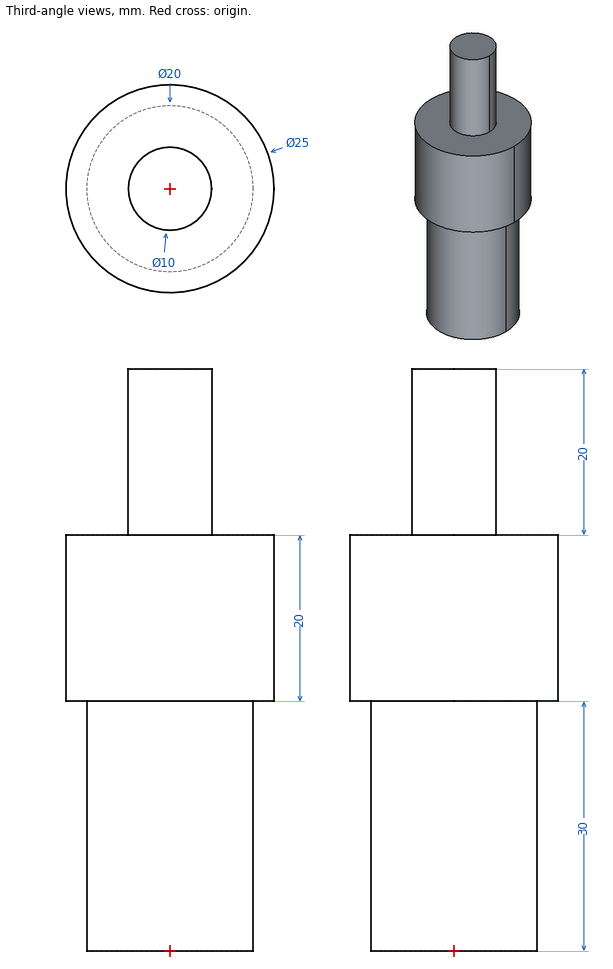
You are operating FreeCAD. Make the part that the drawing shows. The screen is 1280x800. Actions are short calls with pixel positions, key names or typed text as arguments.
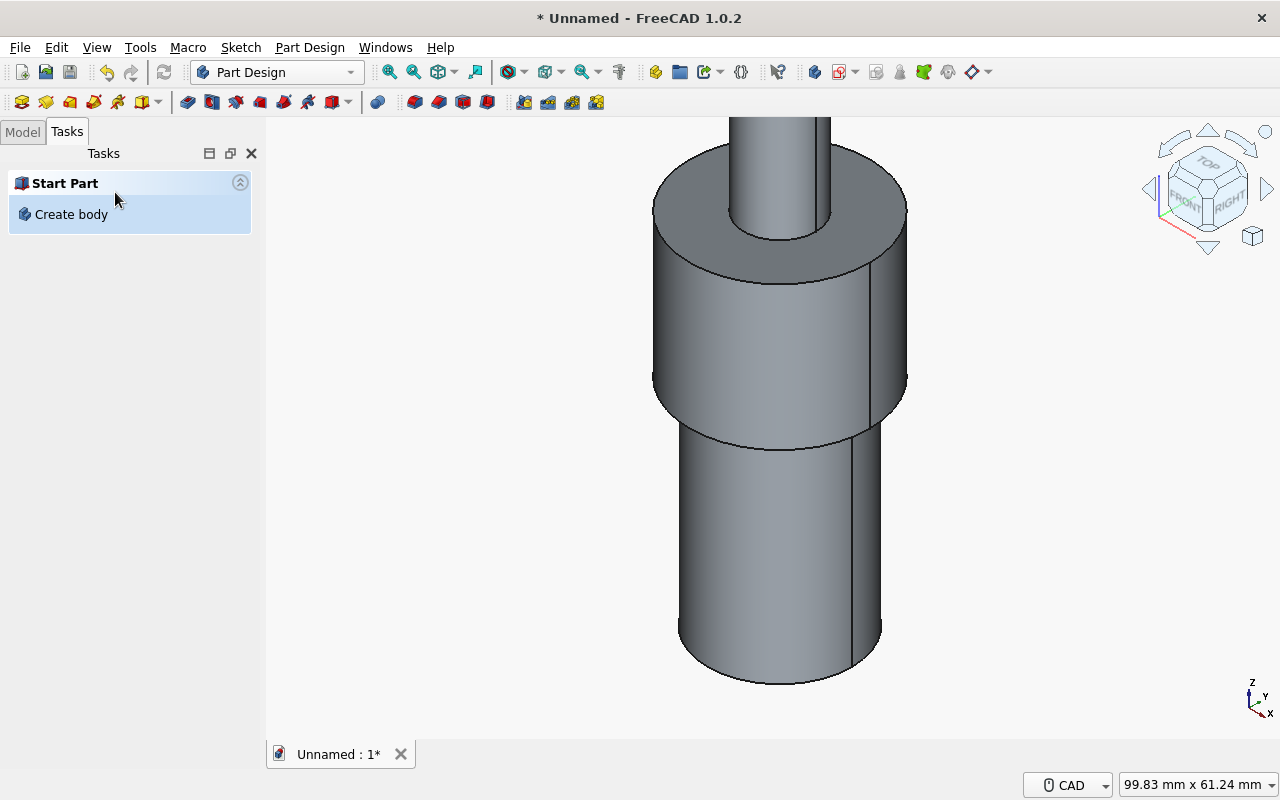
key(v)
key(f)